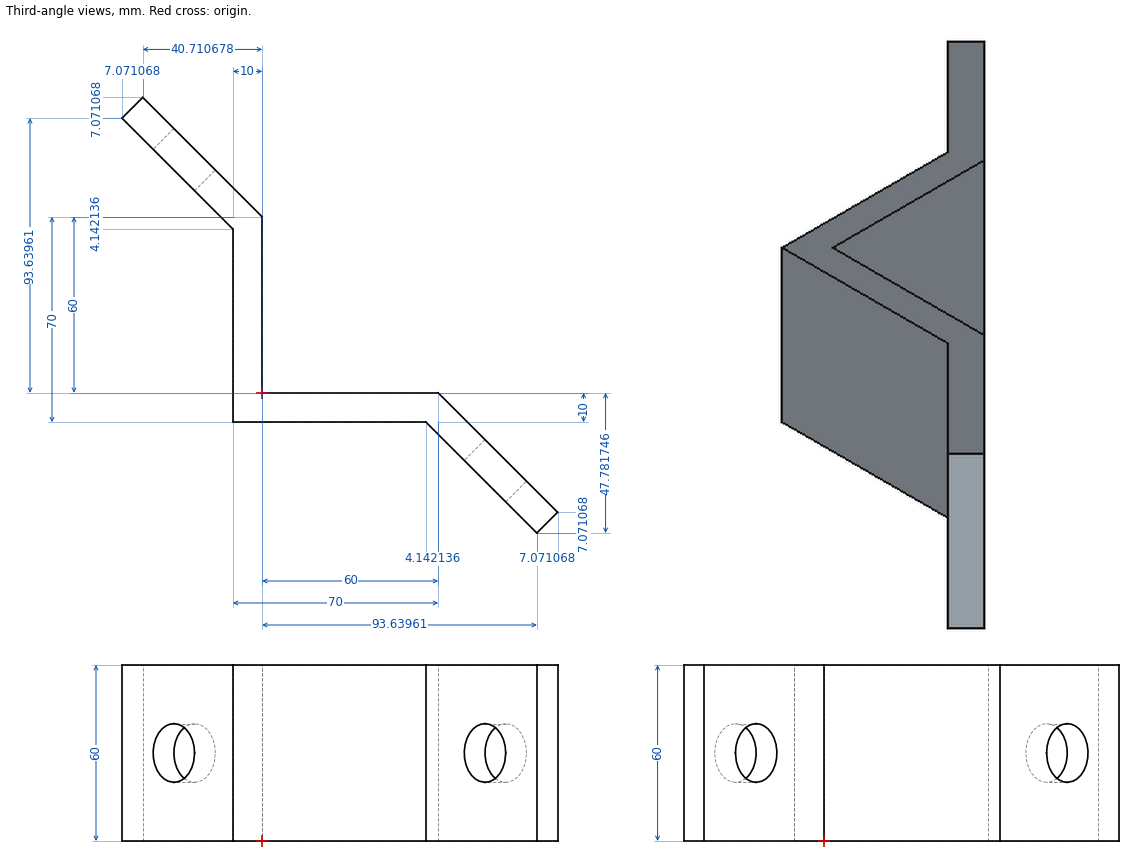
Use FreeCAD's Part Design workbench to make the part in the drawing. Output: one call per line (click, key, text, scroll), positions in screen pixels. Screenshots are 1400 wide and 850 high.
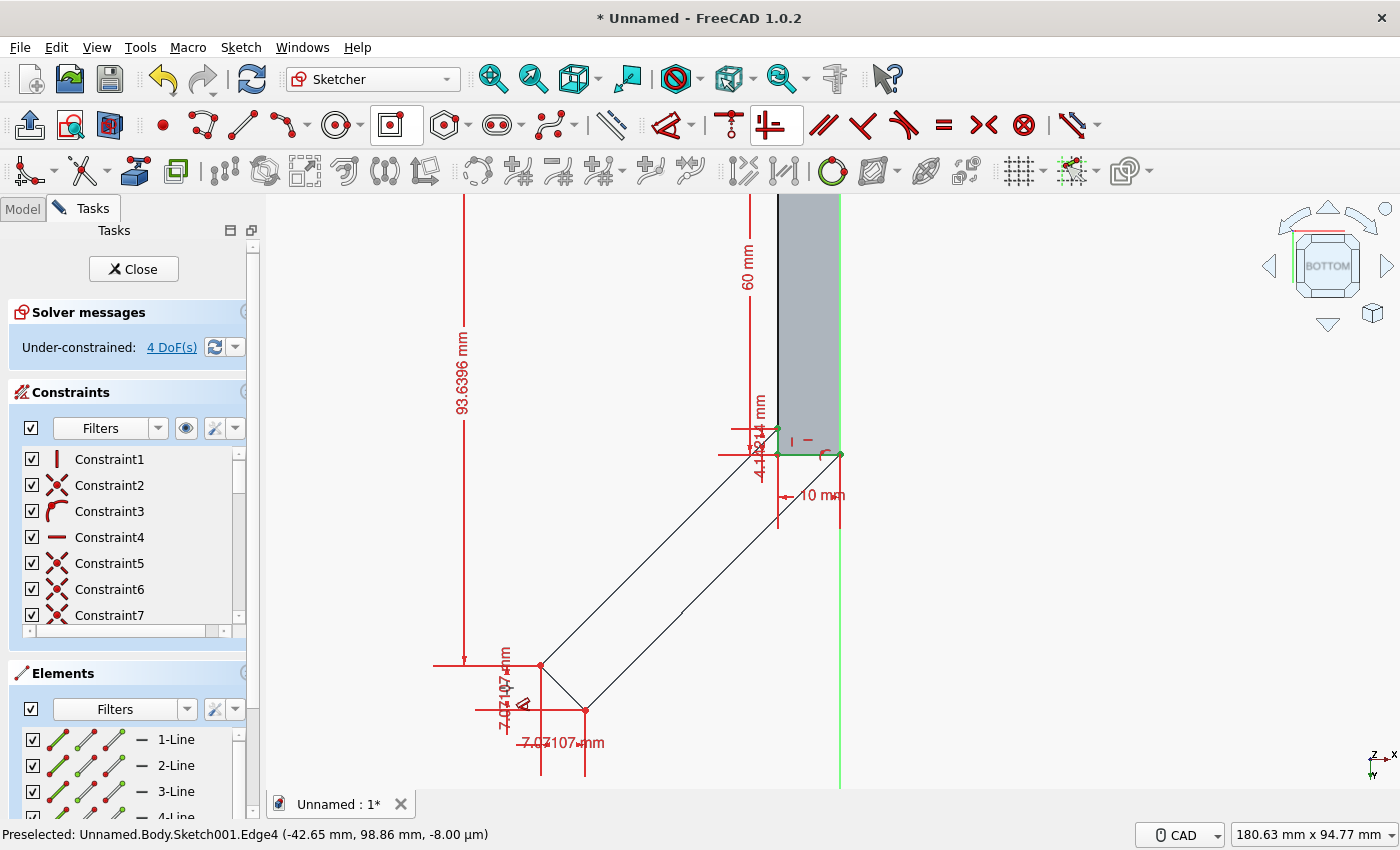
scroll(567, 693, down, 4)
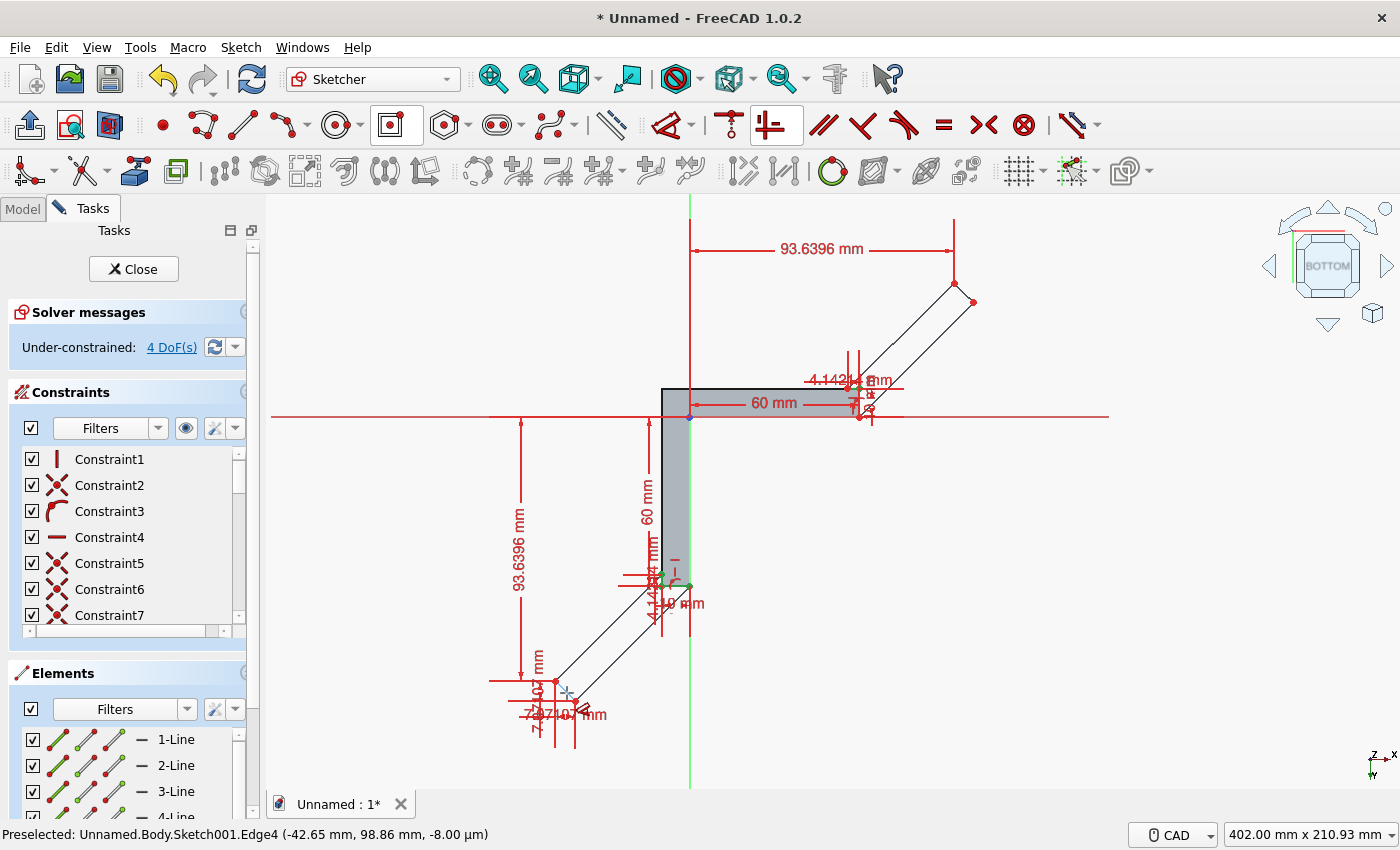
scroll(960, 289, up, 4)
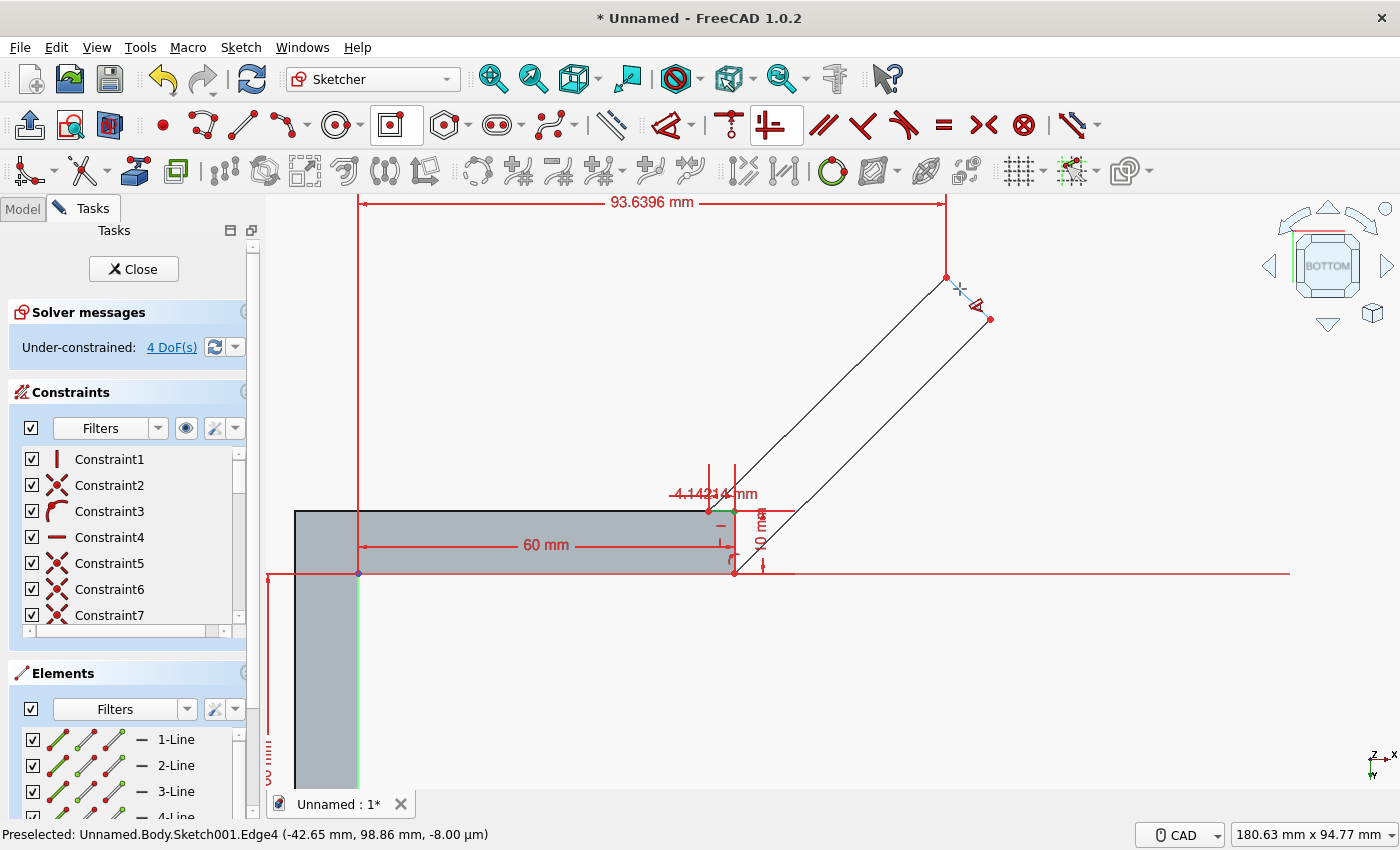
click(959, 290)
click(968, 243)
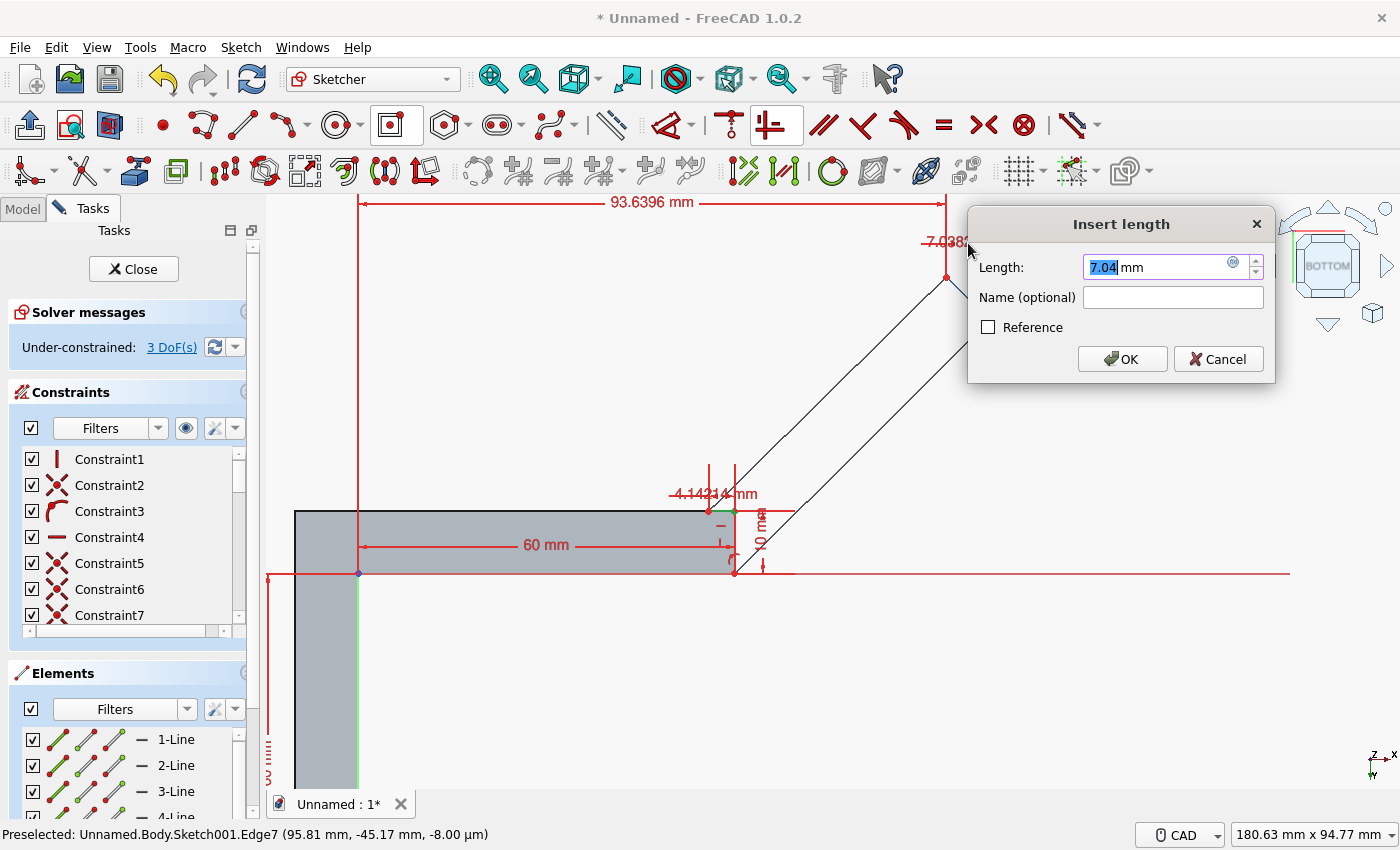
text(7.071068)
key(Return)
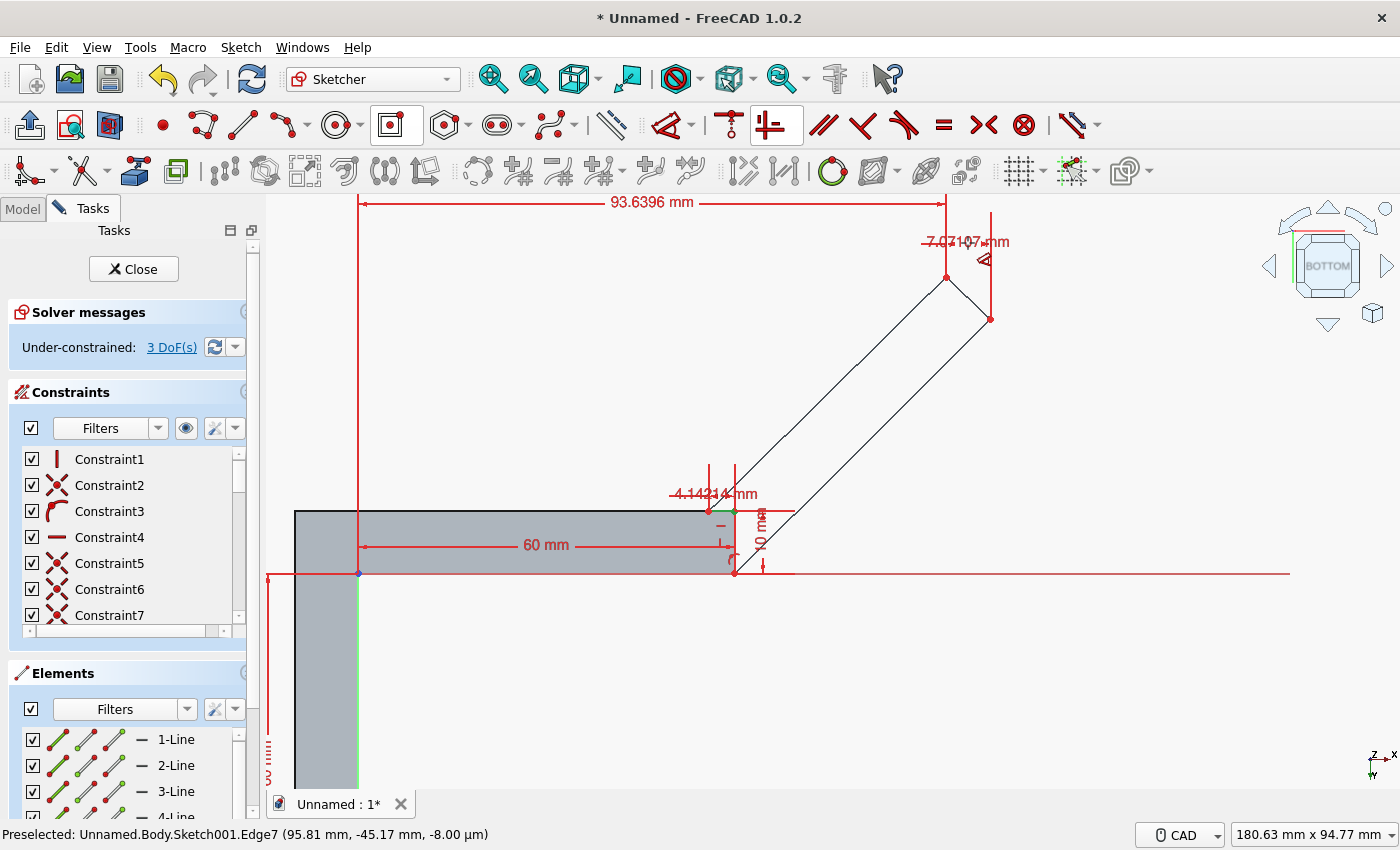
click(959, 290)
click(1025, 298)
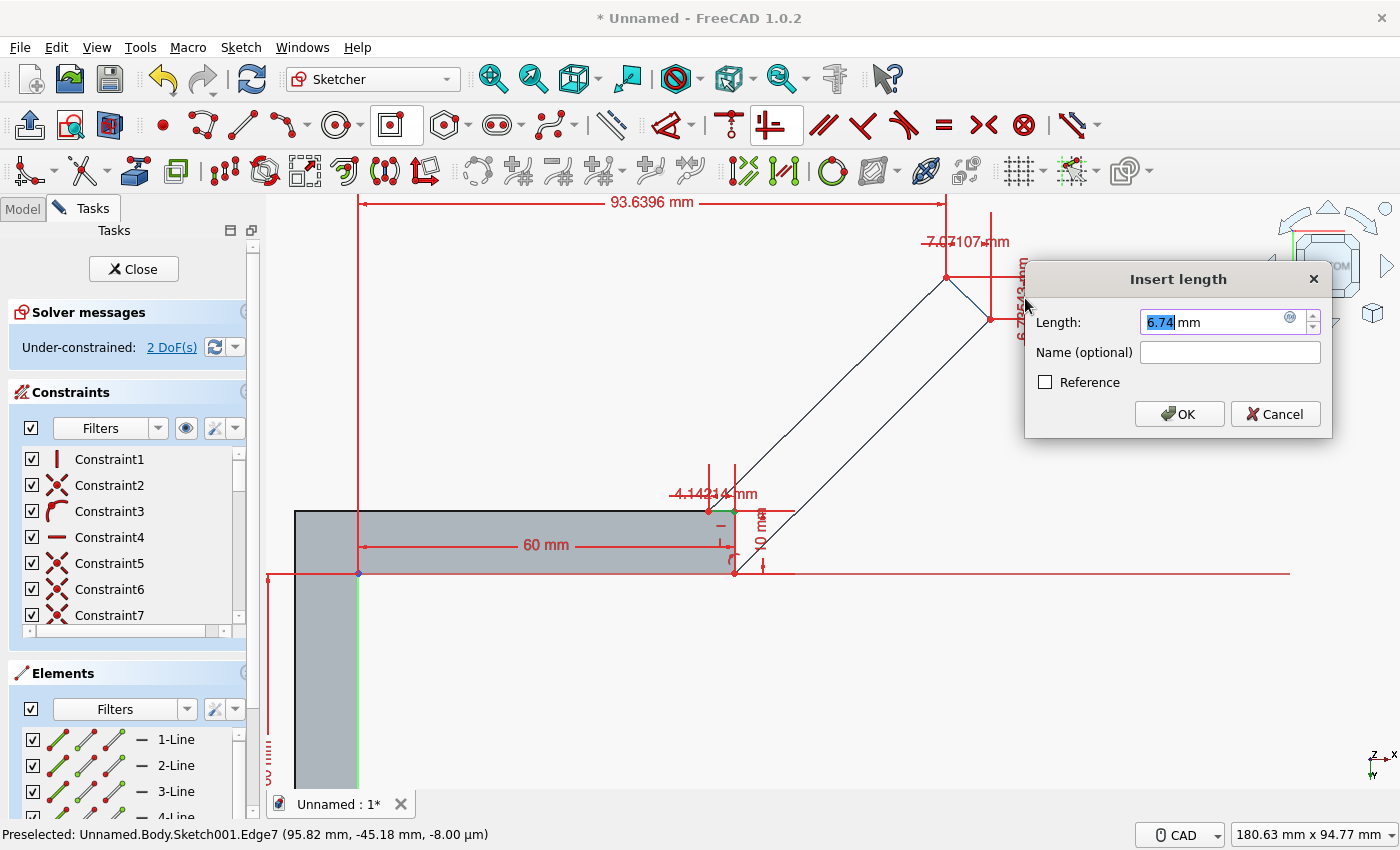
text(7.071068)
key(Return)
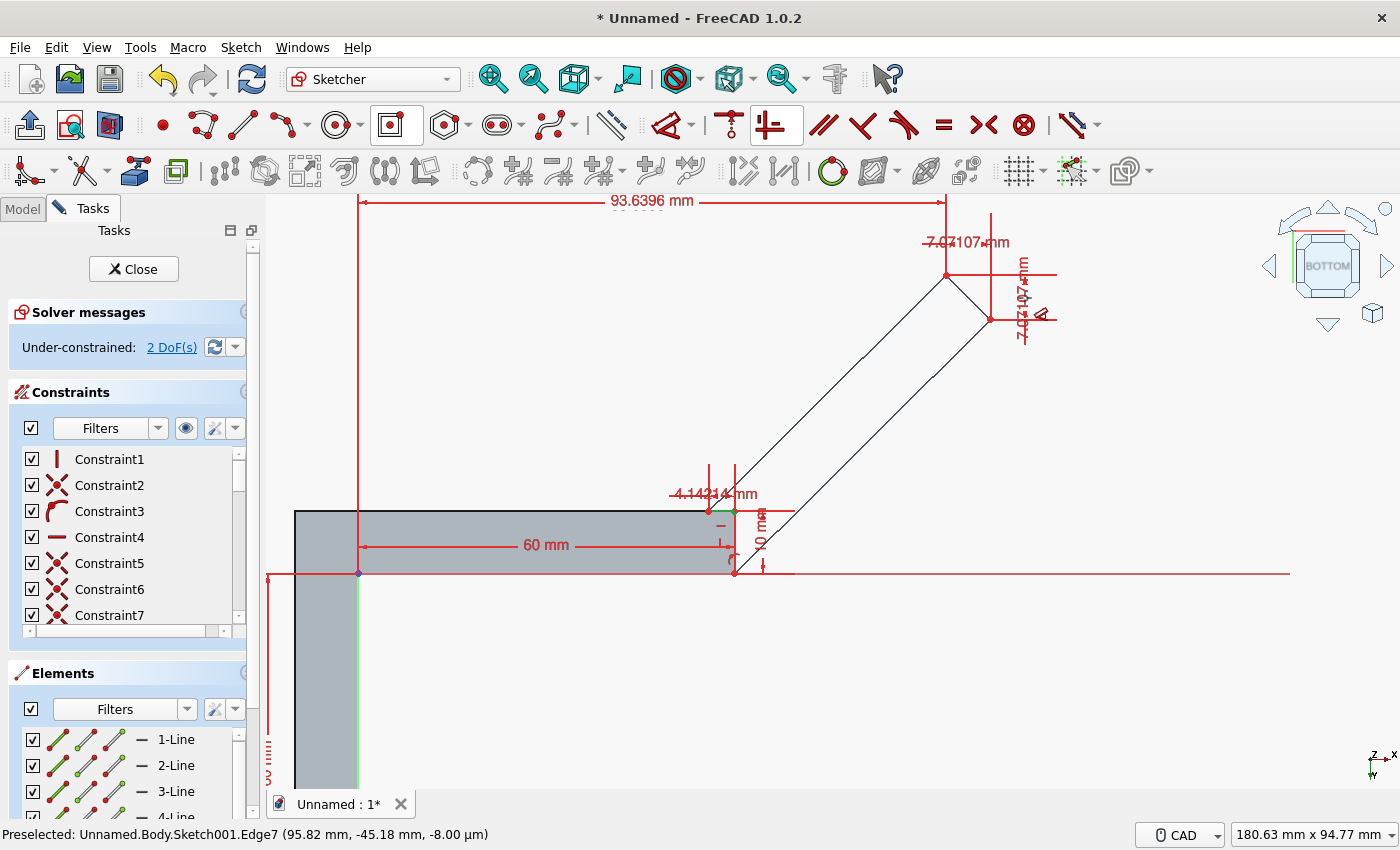
scroll(960, 289, down, 4)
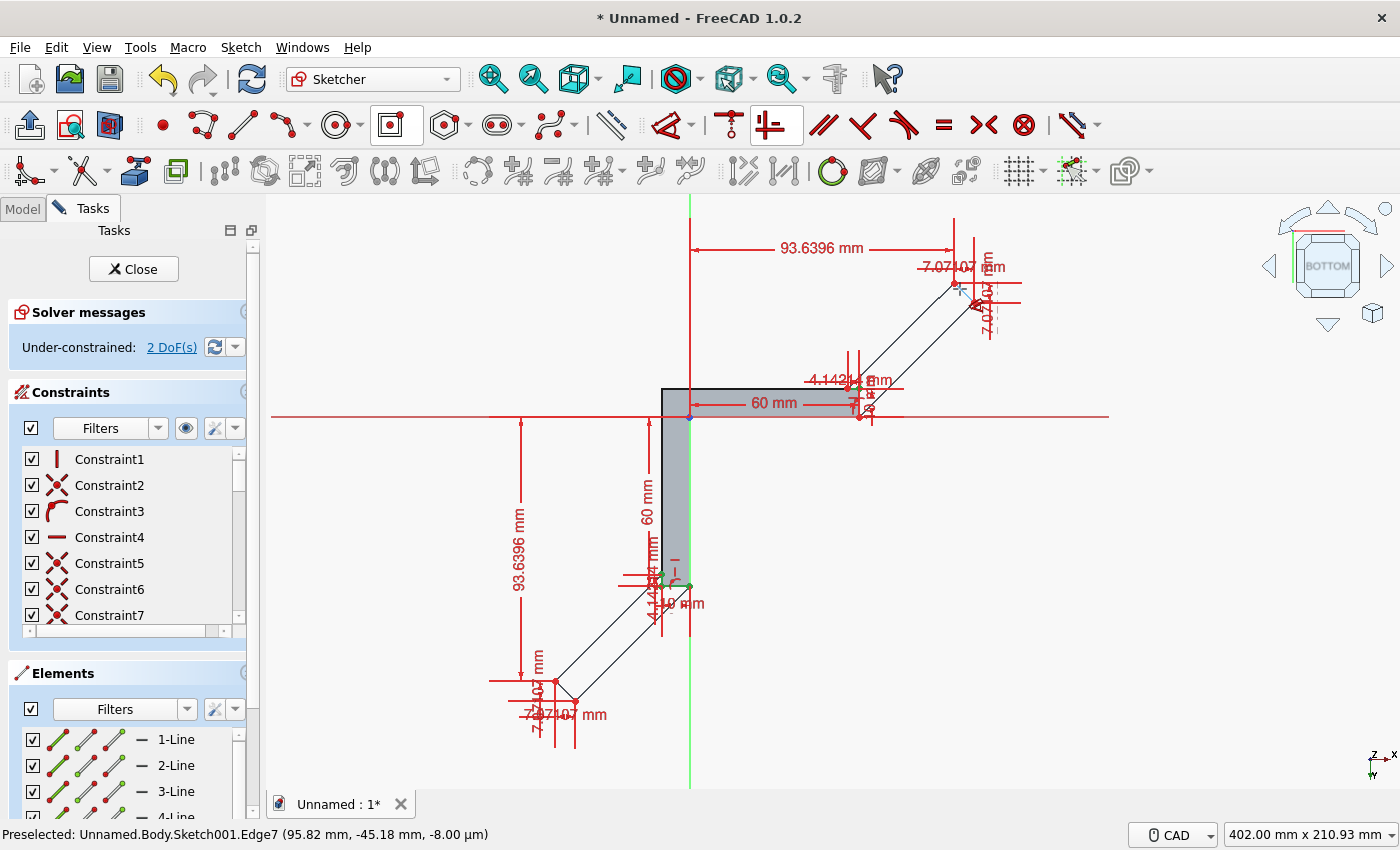
click(575, 701)
click(659, 735)